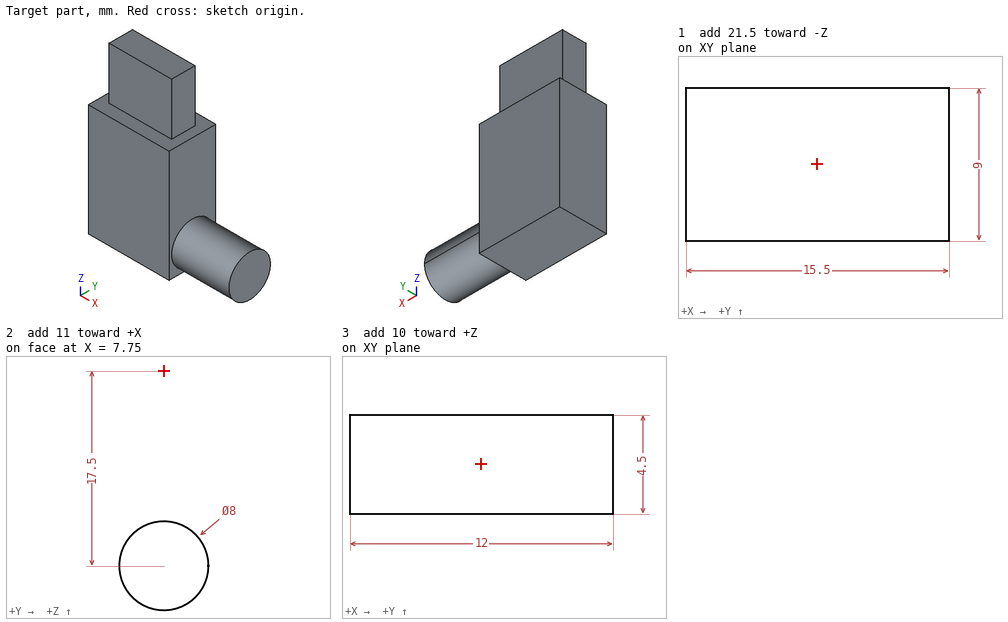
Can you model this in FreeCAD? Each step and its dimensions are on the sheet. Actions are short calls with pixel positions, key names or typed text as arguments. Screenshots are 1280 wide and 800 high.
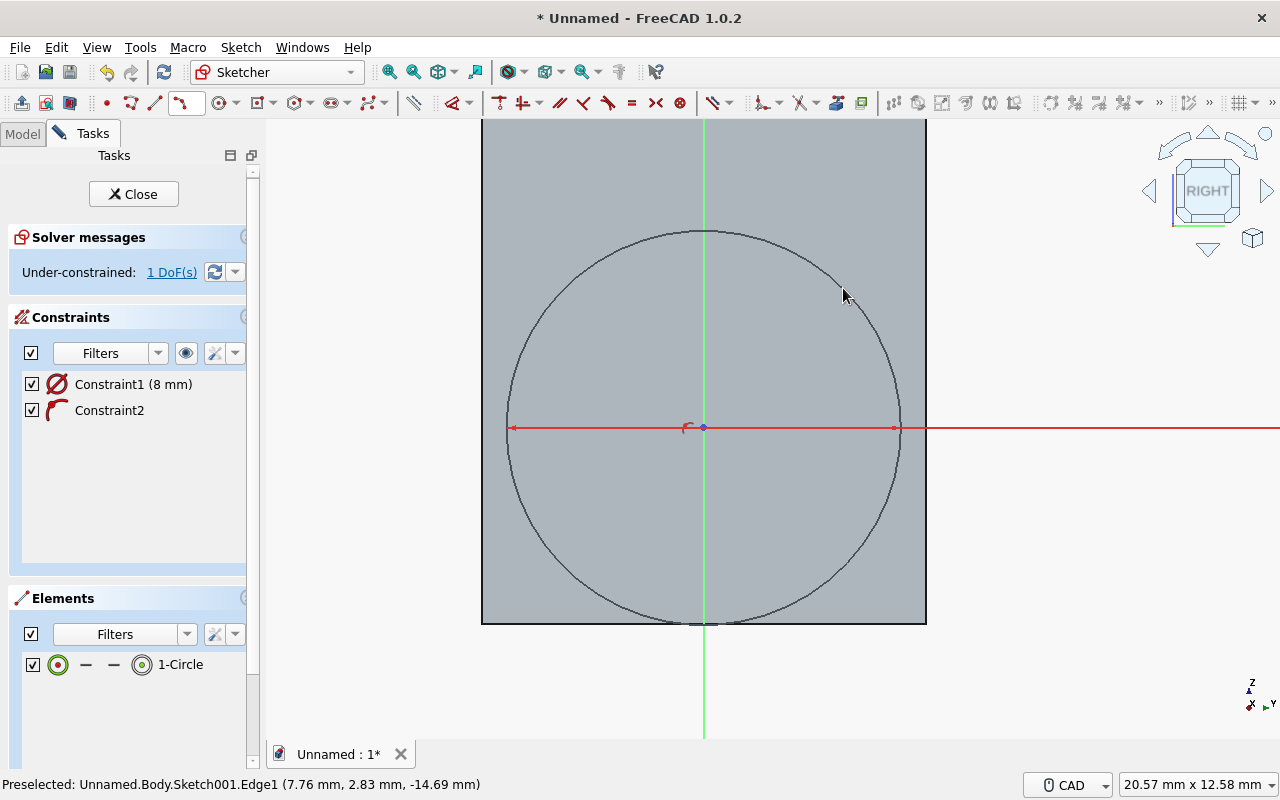
click(452, 104)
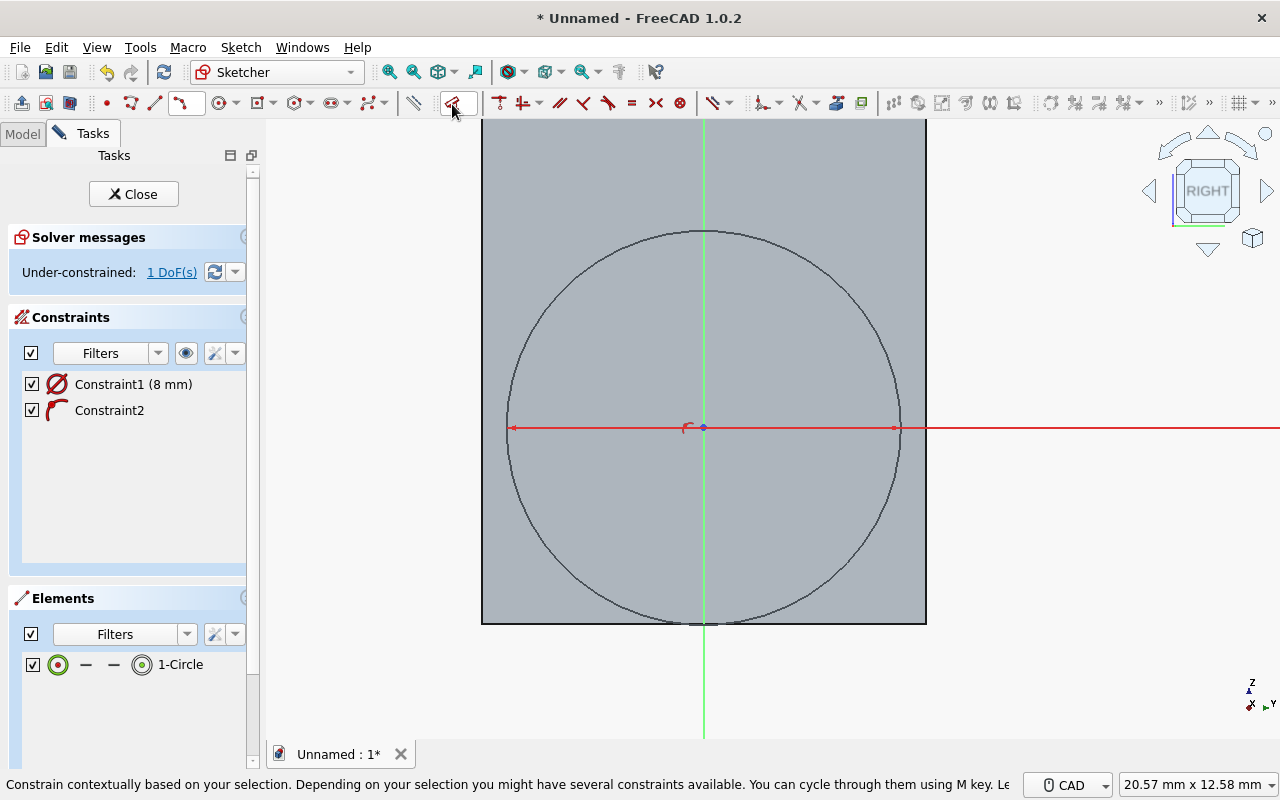
click(704, 428)
click(738, 287)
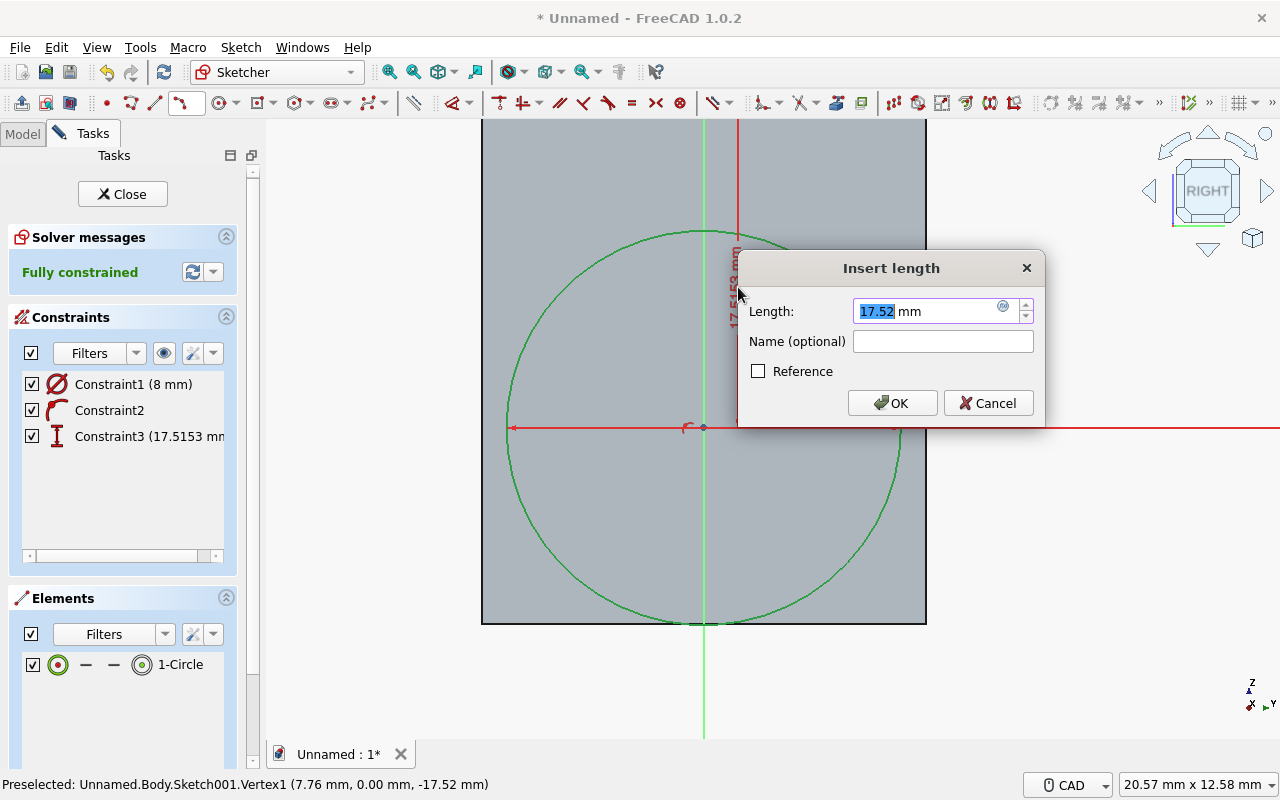
text(17.5)
key(Return)
key(Escape)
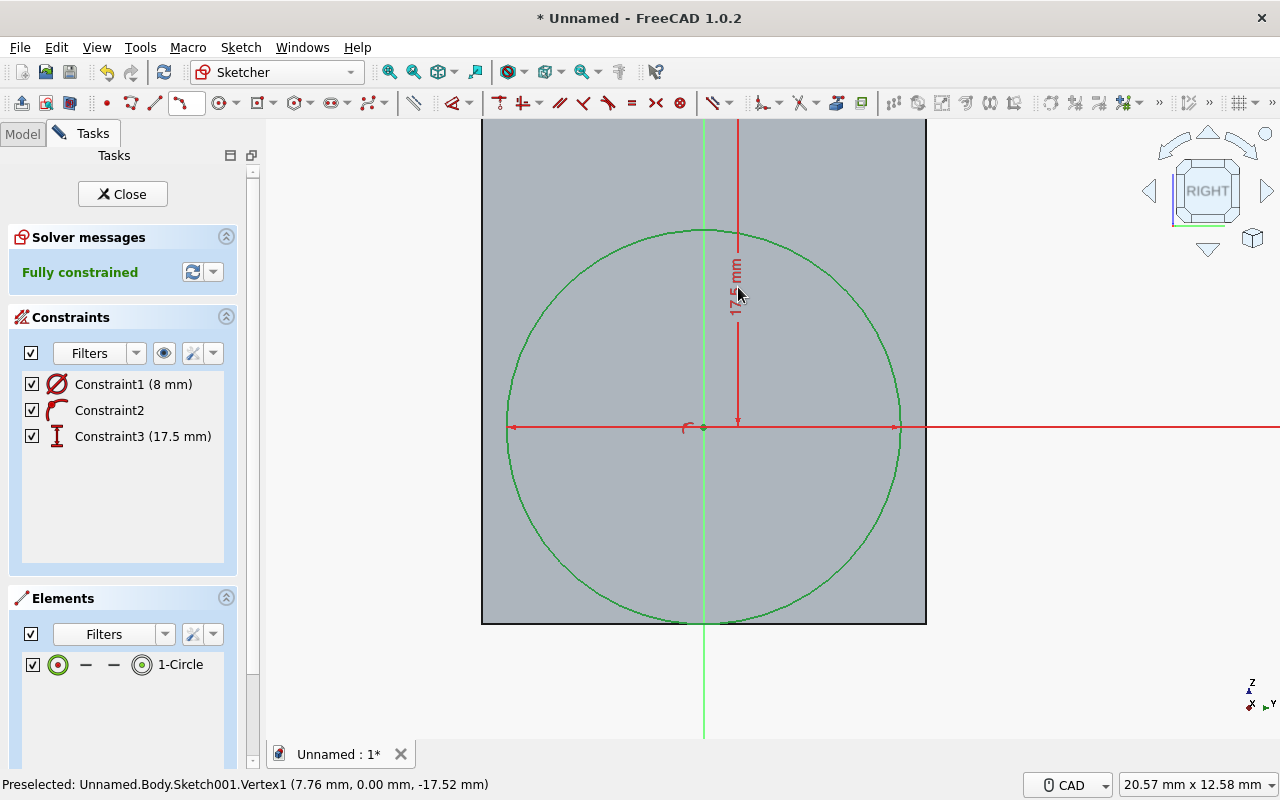
click(123, 194)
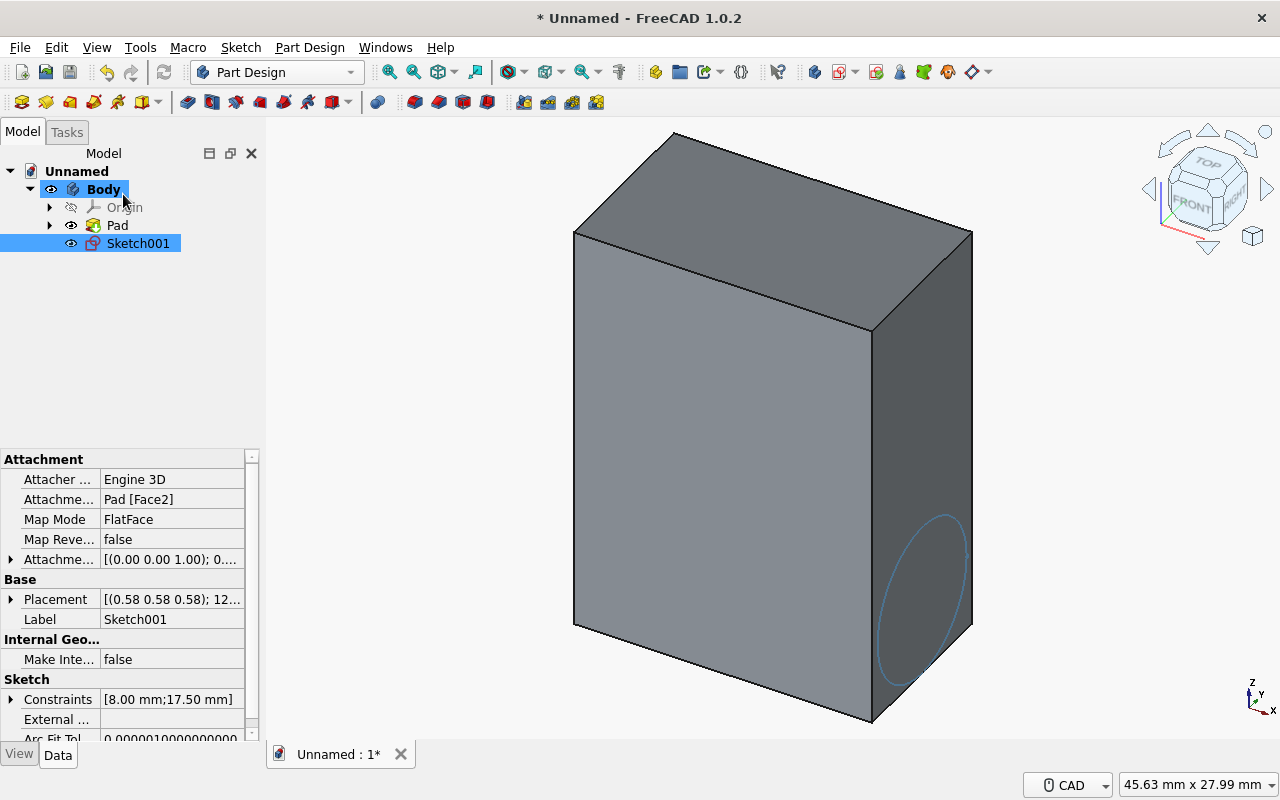
click(22, 102)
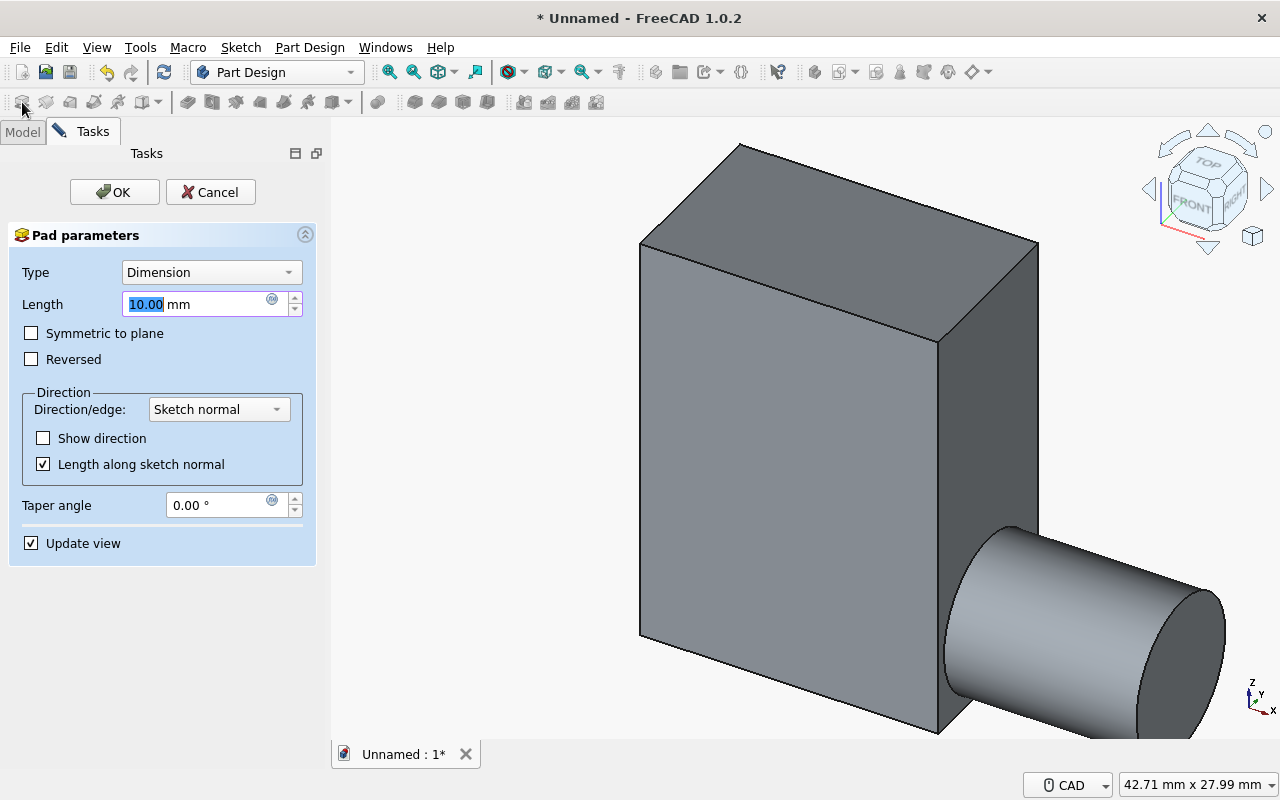
text(11)
key(Tab)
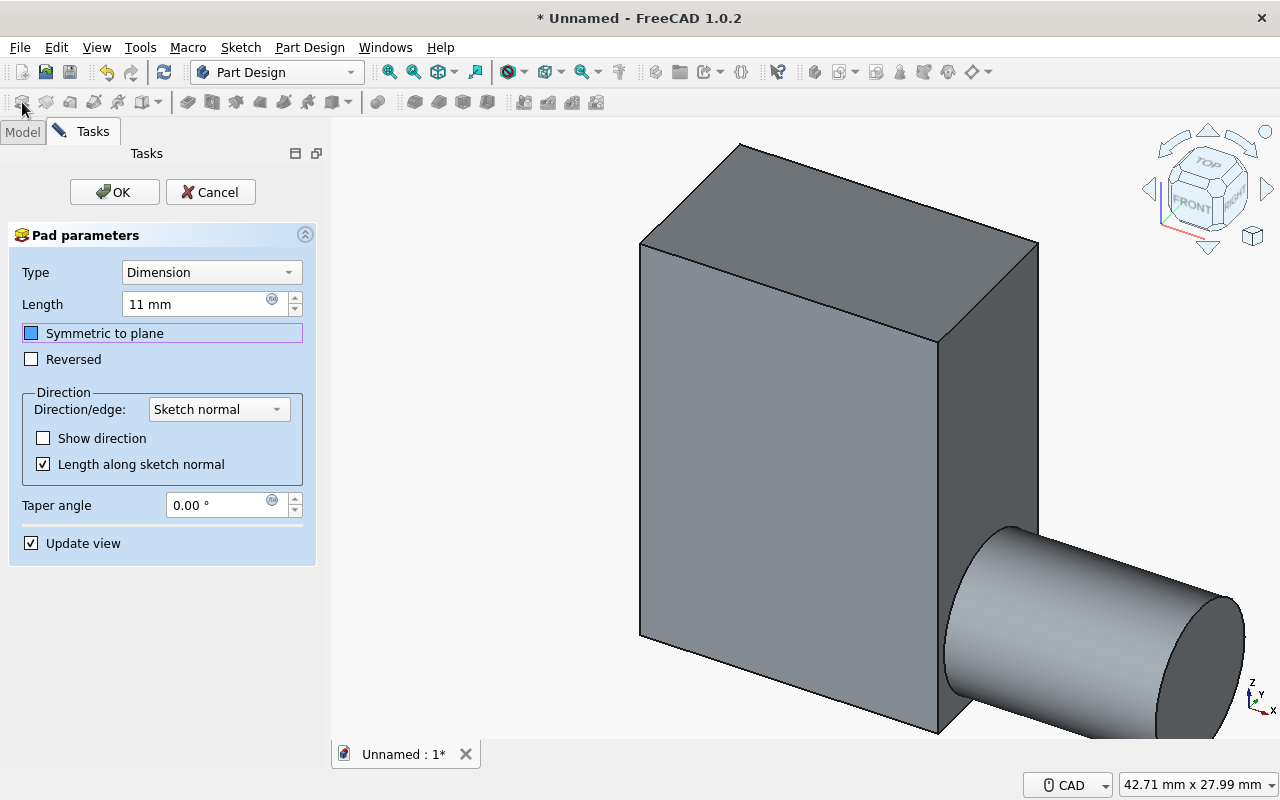
click(115, 192)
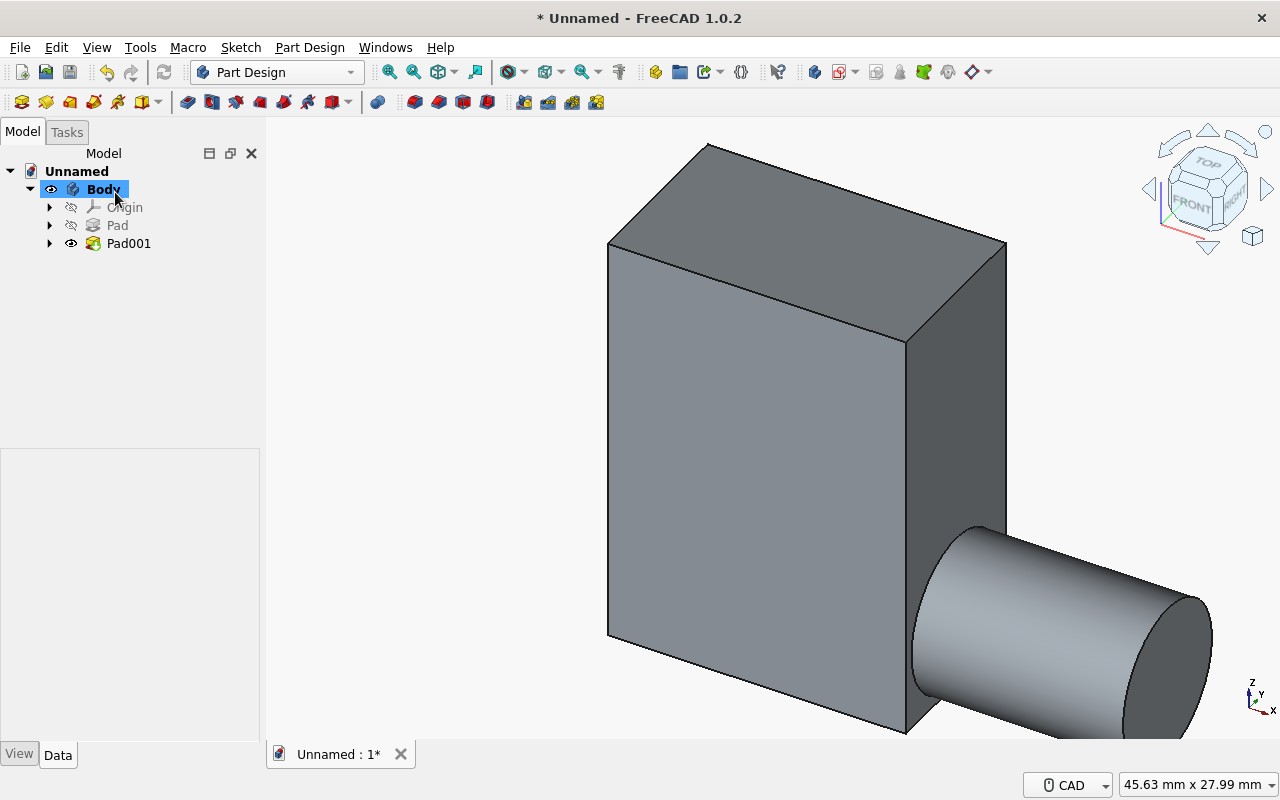
click(390, 72)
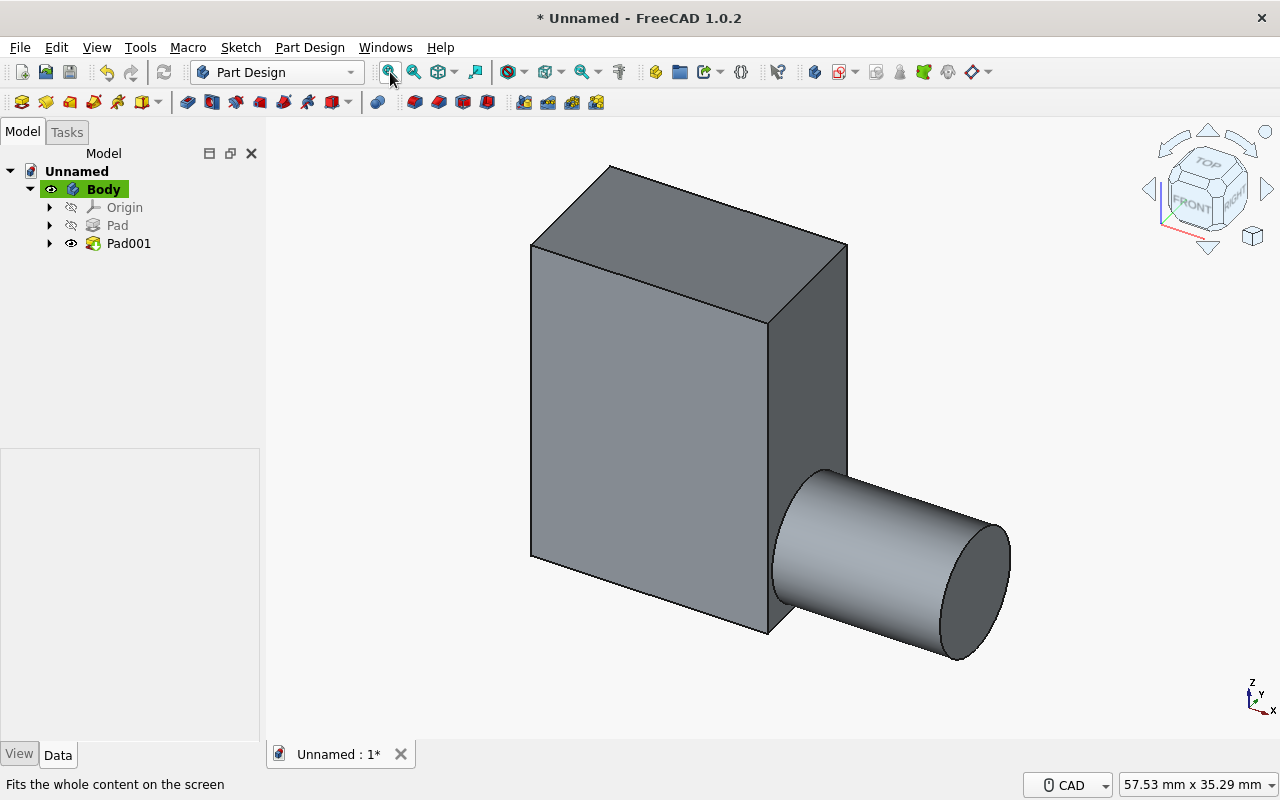
click(840, 72)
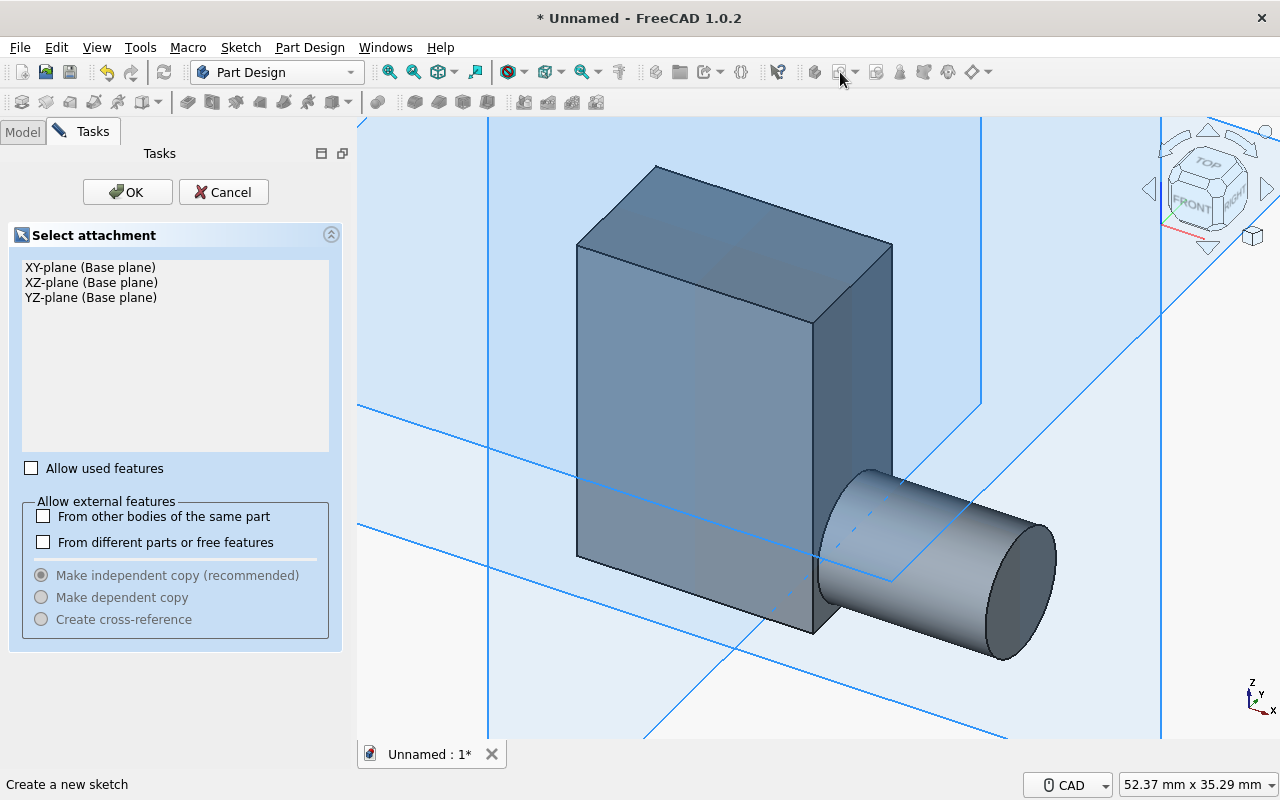
click(82, 268)